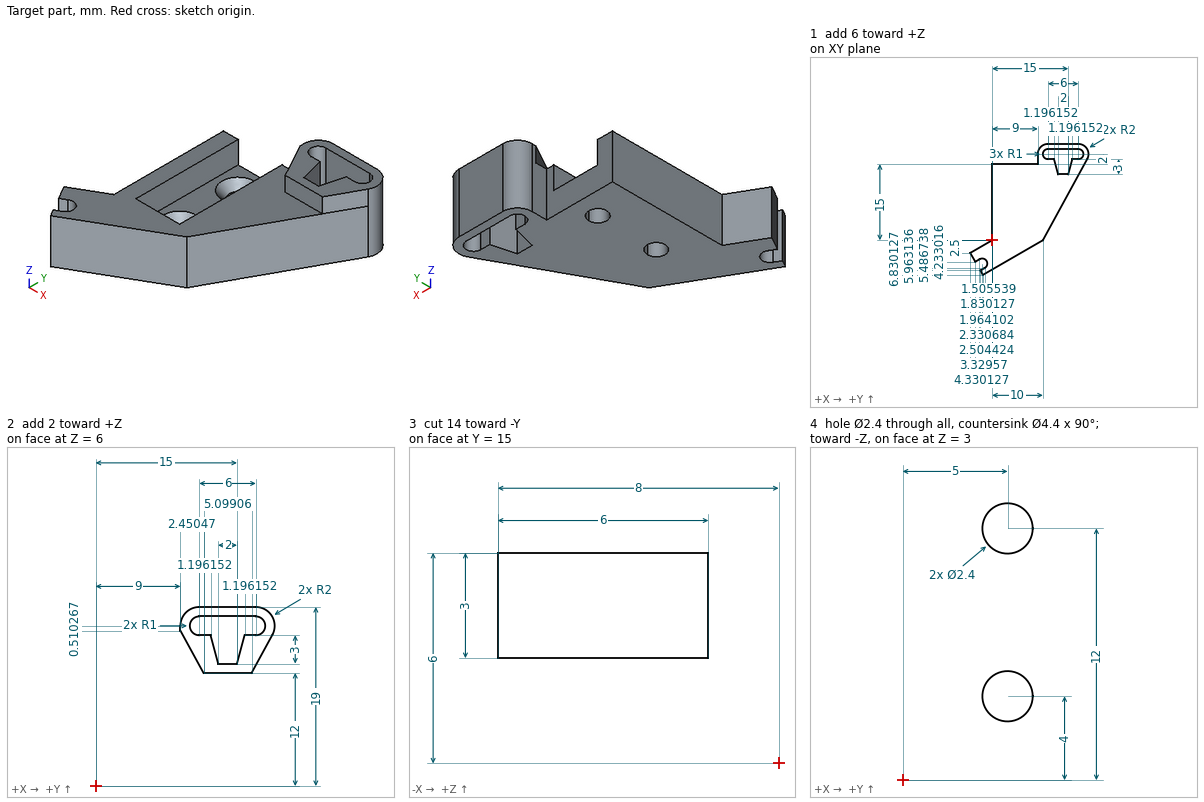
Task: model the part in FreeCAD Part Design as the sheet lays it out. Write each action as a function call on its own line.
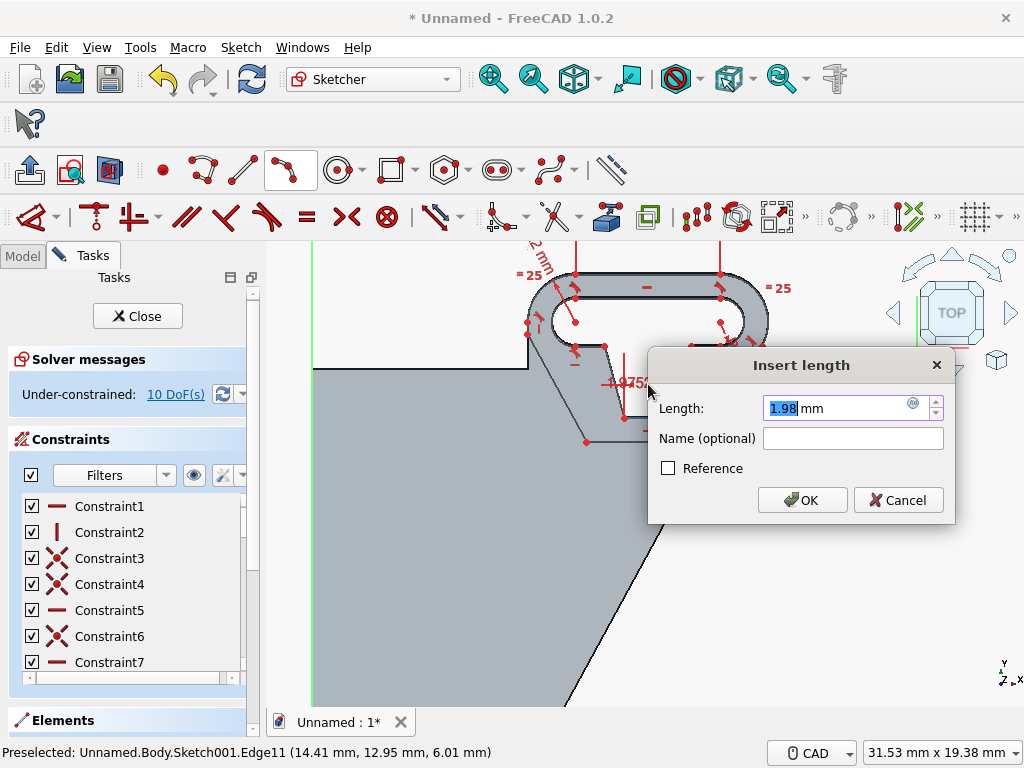
text(2)
key(Return)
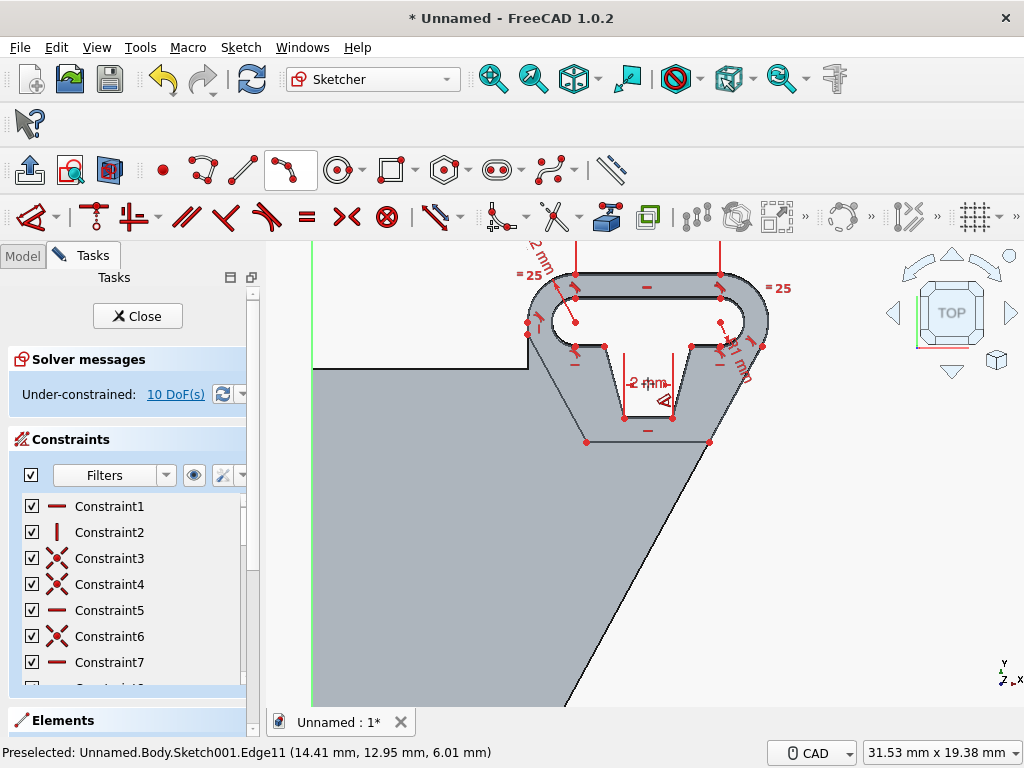
click(528, 323)
click(420, 289)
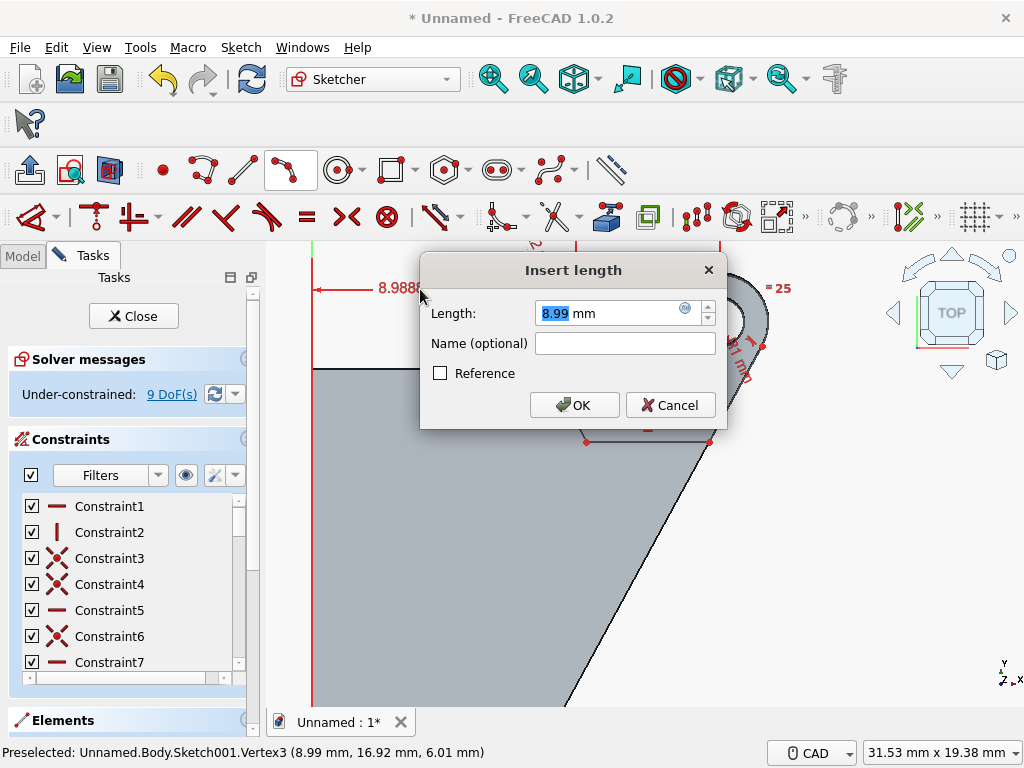
text(9)
key(Return)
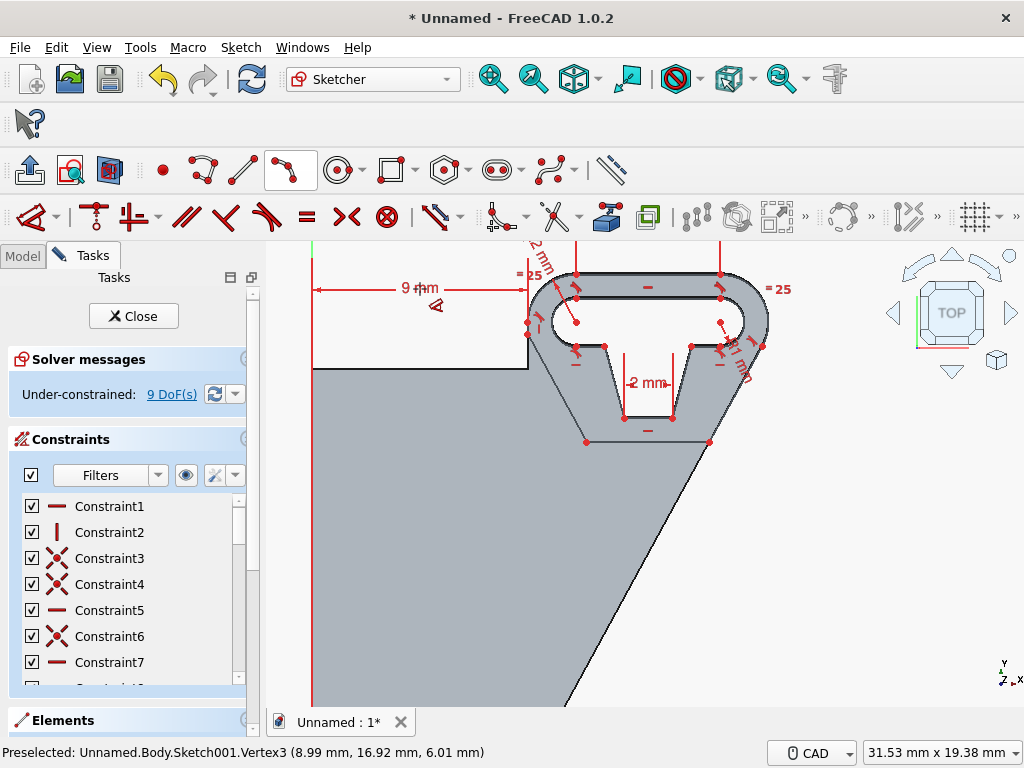
click(686, 368)
click(726, 383)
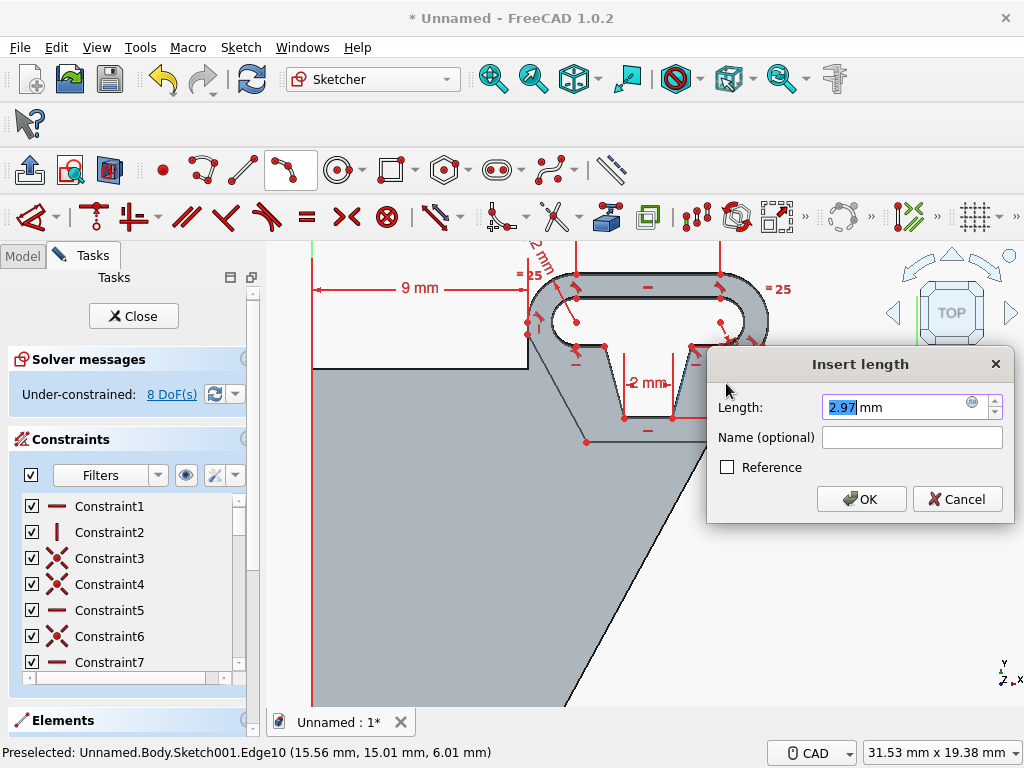
text(3)
key(Return)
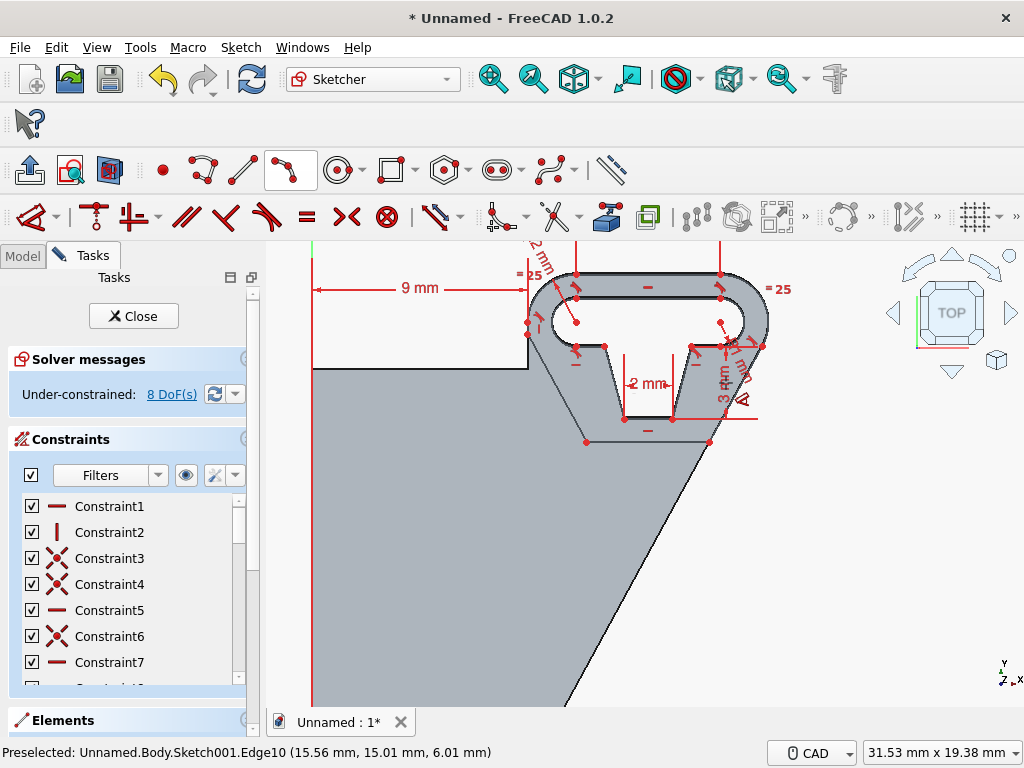
click(720, 275)
click(754, 477)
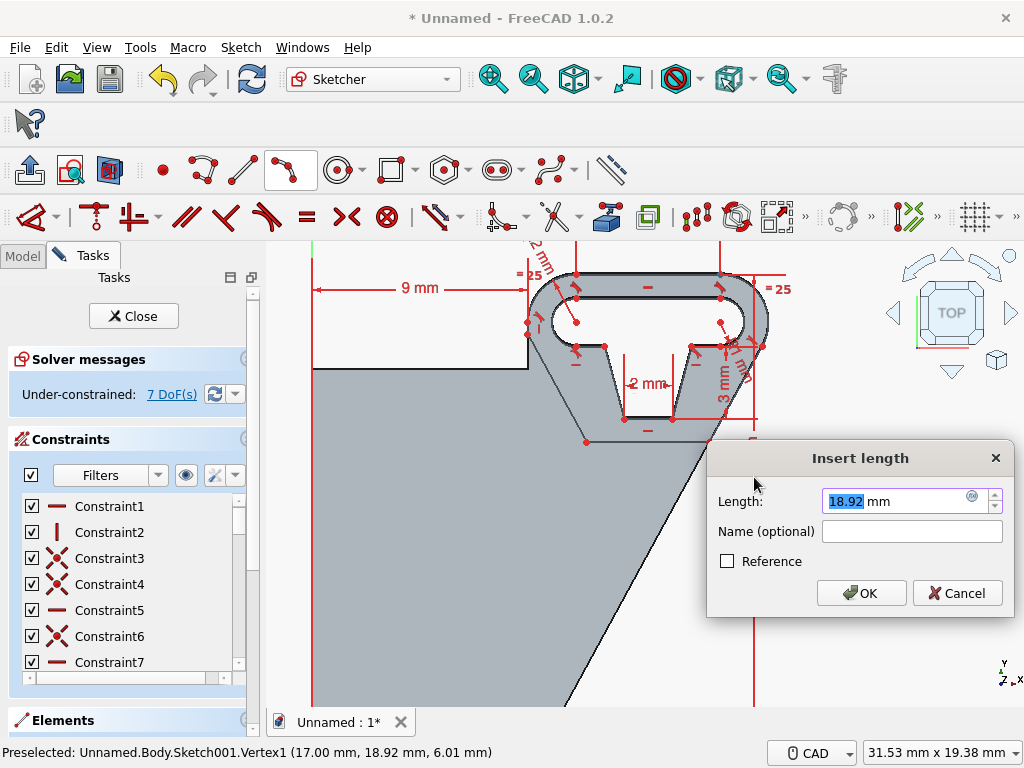
text(19)
key(Return)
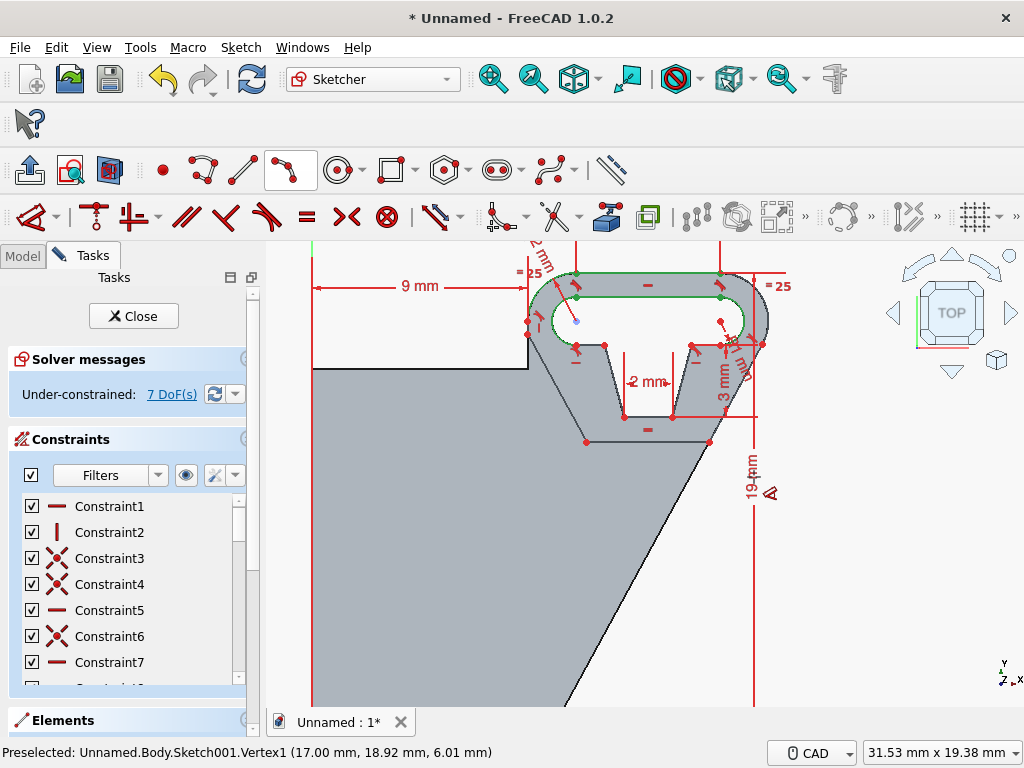
click(587, 442)
click(621, 561)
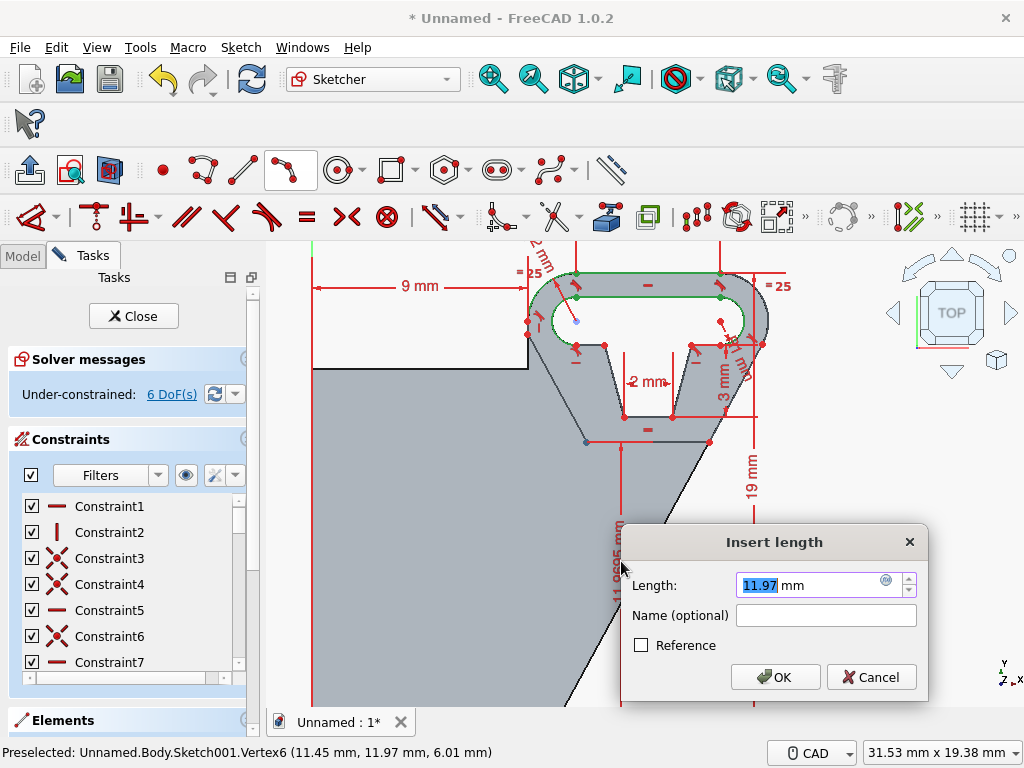
text(12)
key(Return)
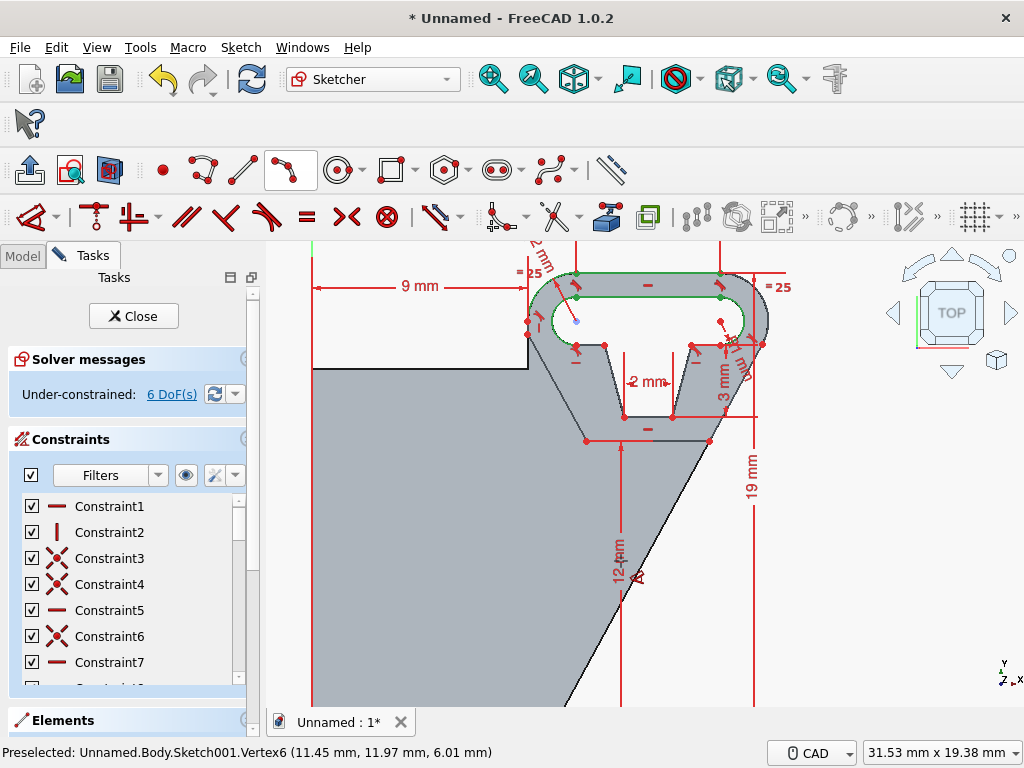
click(673, 417)
click(492, 383)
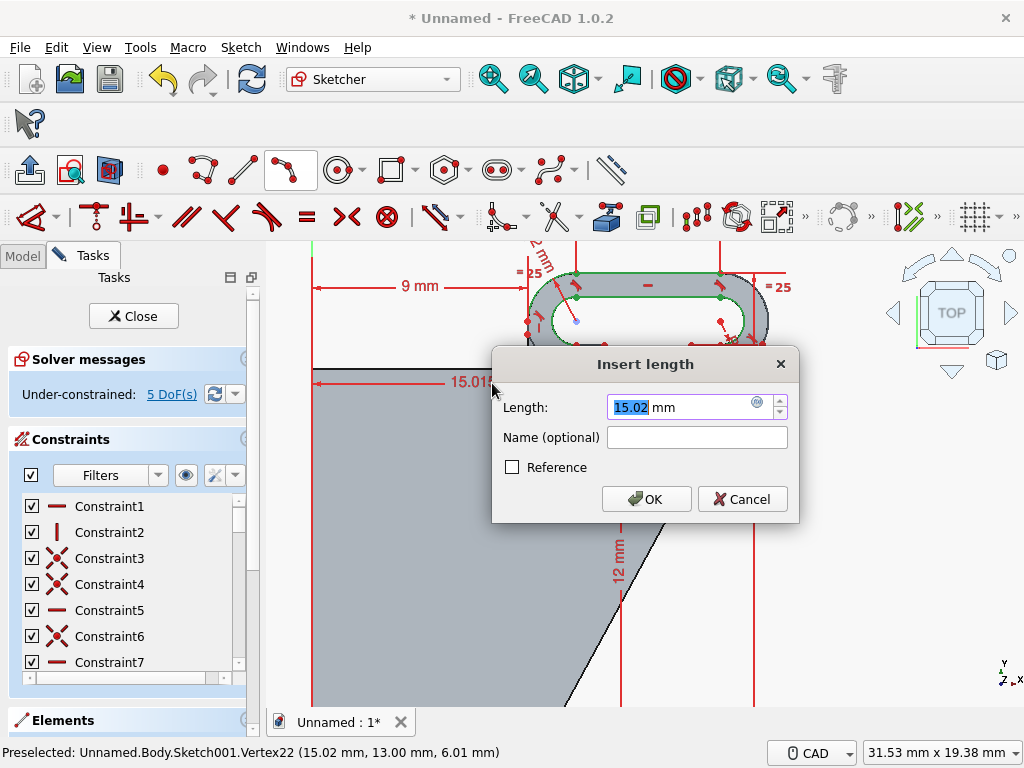
text(15)
key(Return)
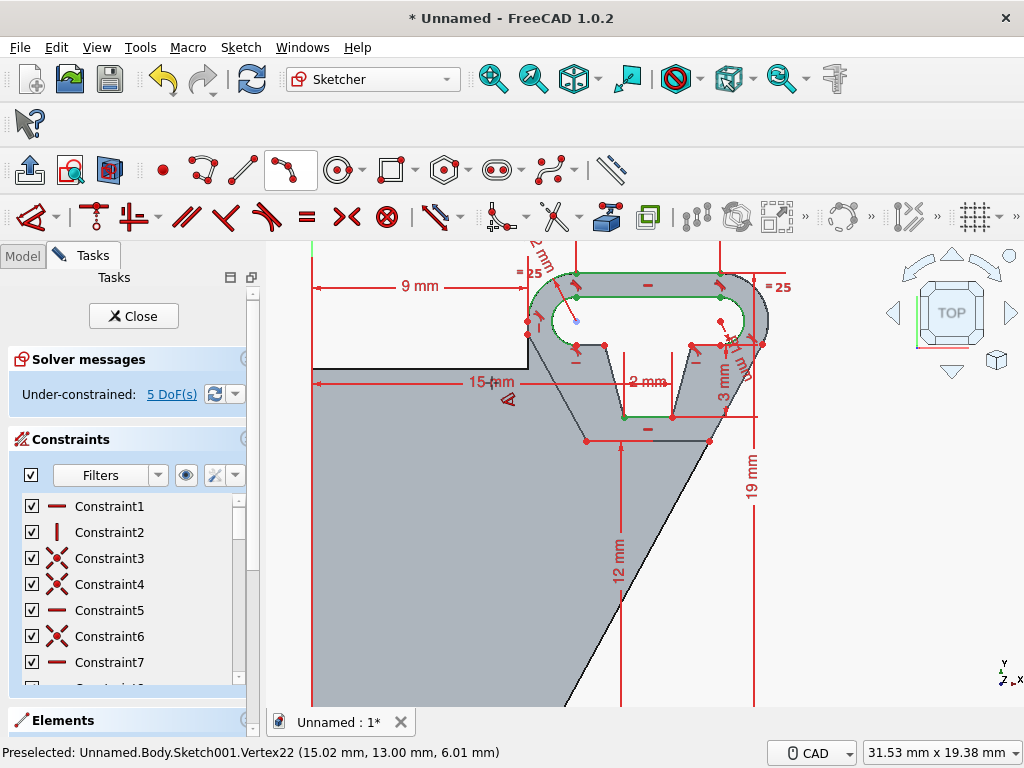
click(624, 441)
click(605, 407)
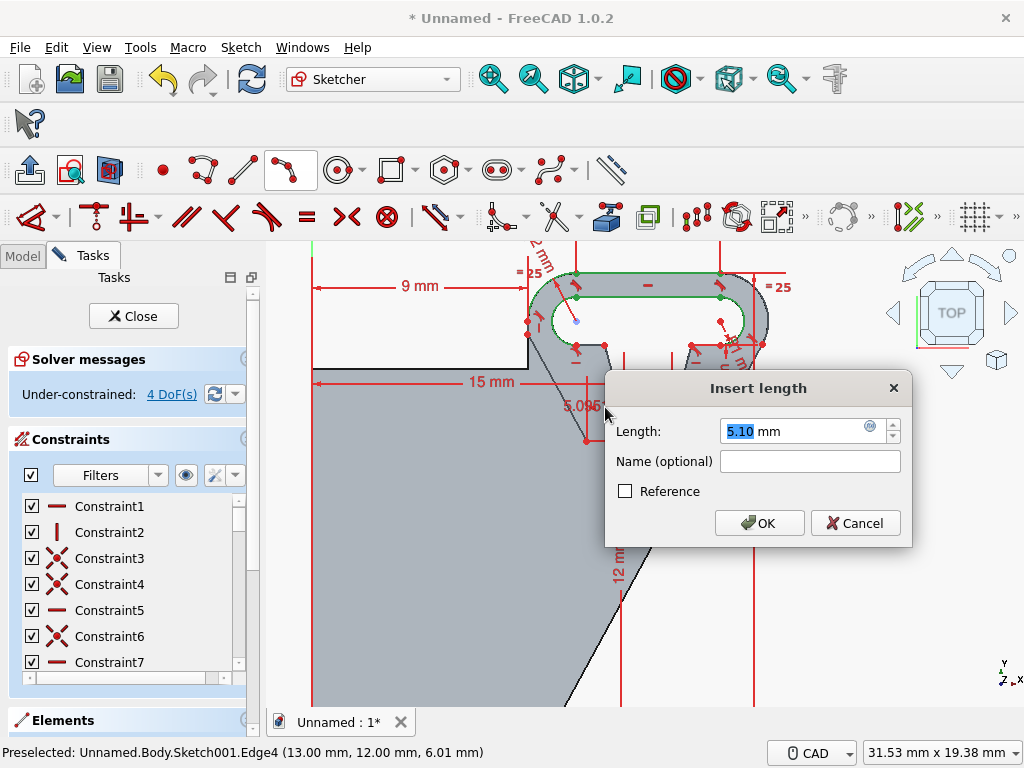
text(5.09906)
key(Return)